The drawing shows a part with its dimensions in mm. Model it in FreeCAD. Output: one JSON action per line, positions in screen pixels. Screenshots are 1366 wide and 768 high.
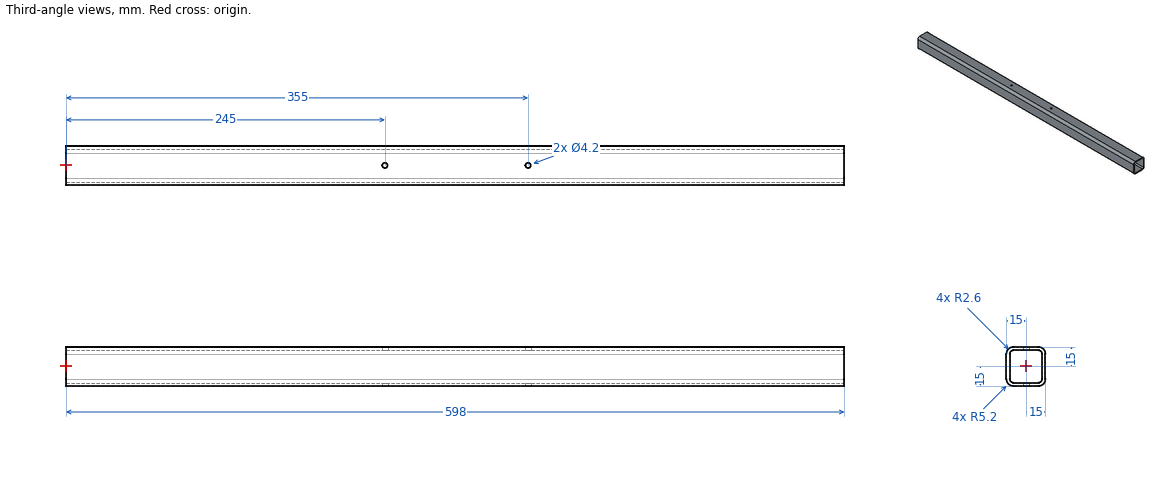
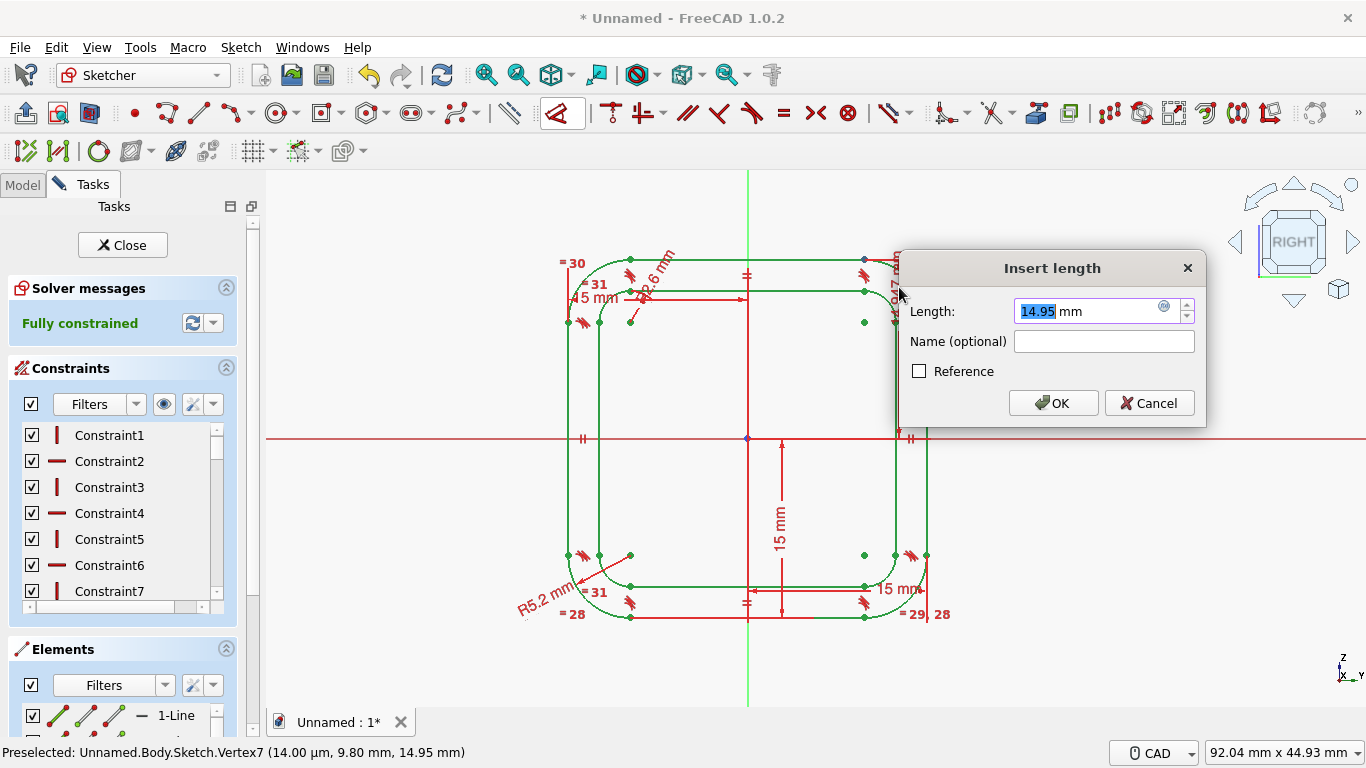
{"action": "type", "text": "15"}
{"action": "key", "text": "Return"}
{"action": "key", "text": "Escape"}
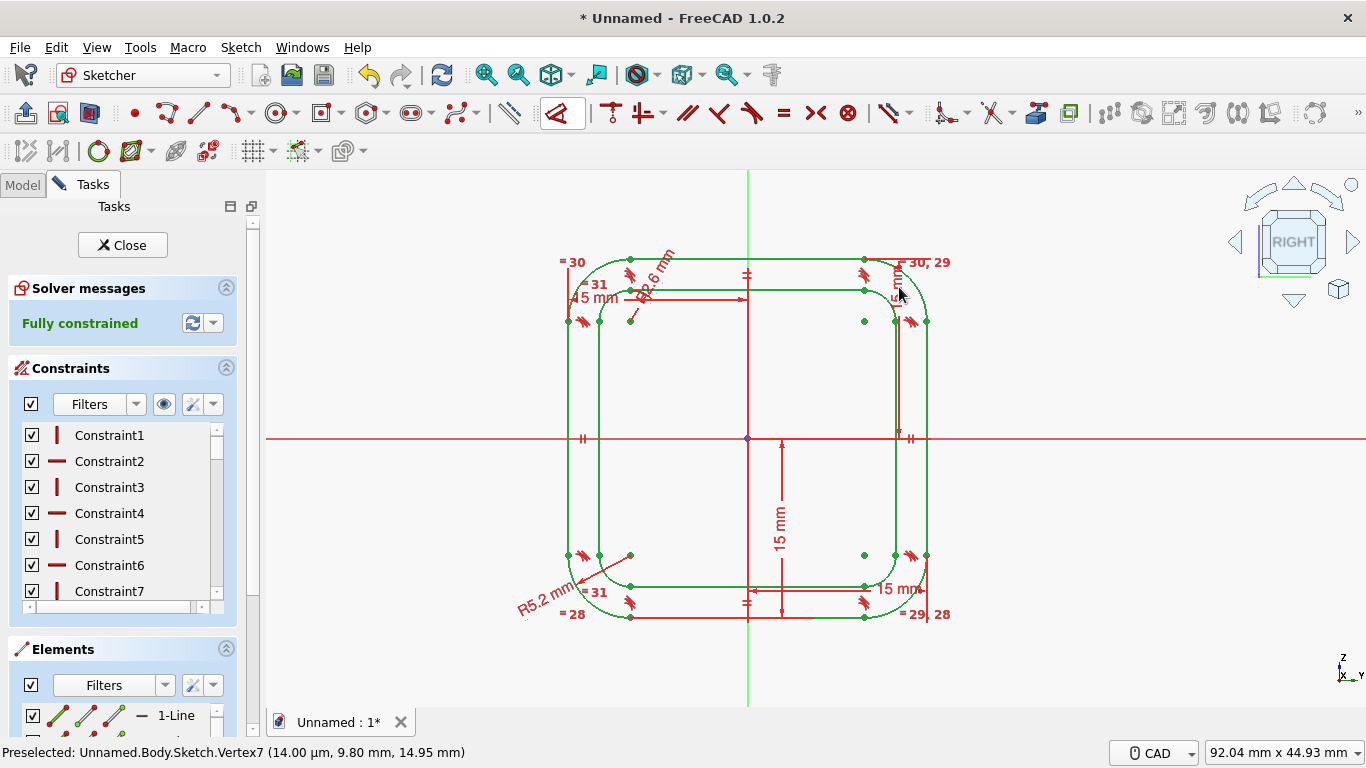
{"action": "left_click", "coordinate": [123, 245]}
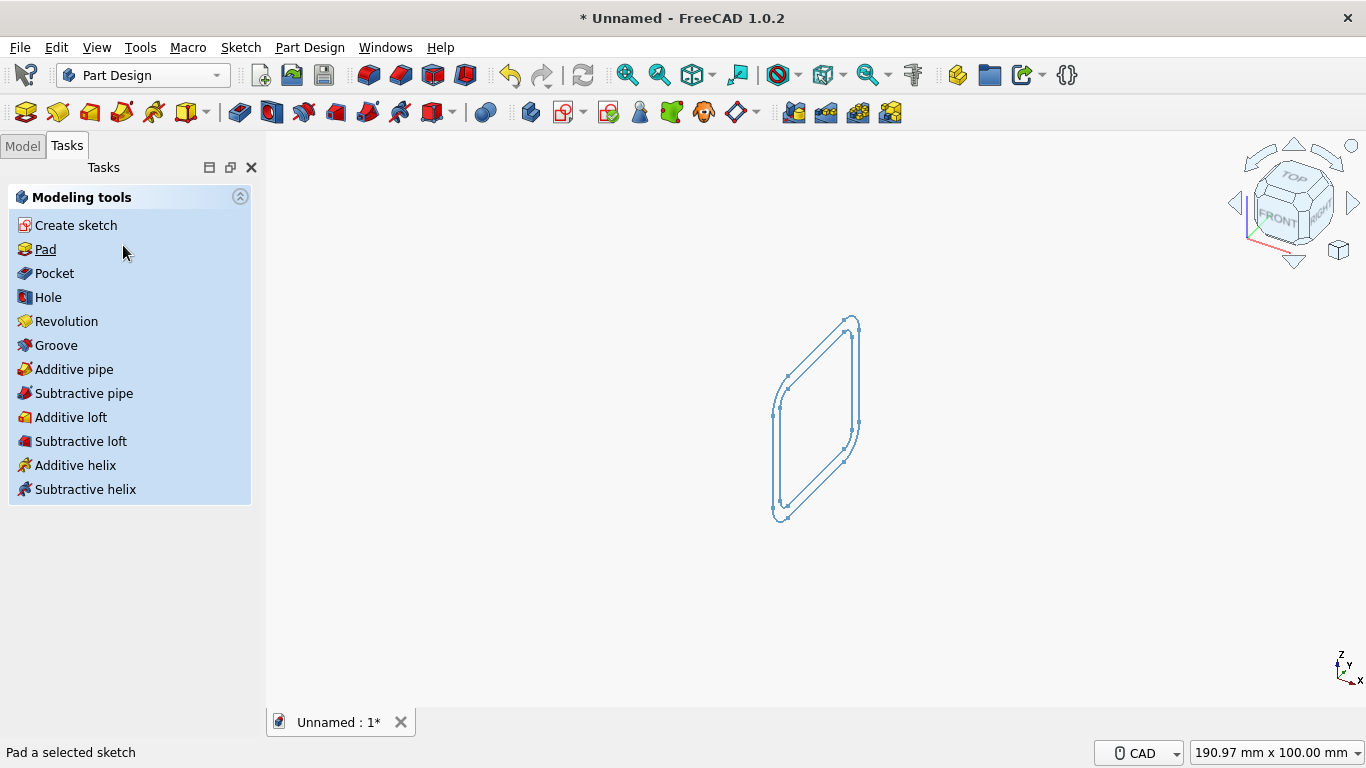
{"action": "left_click", "coordinate": [26, 112]}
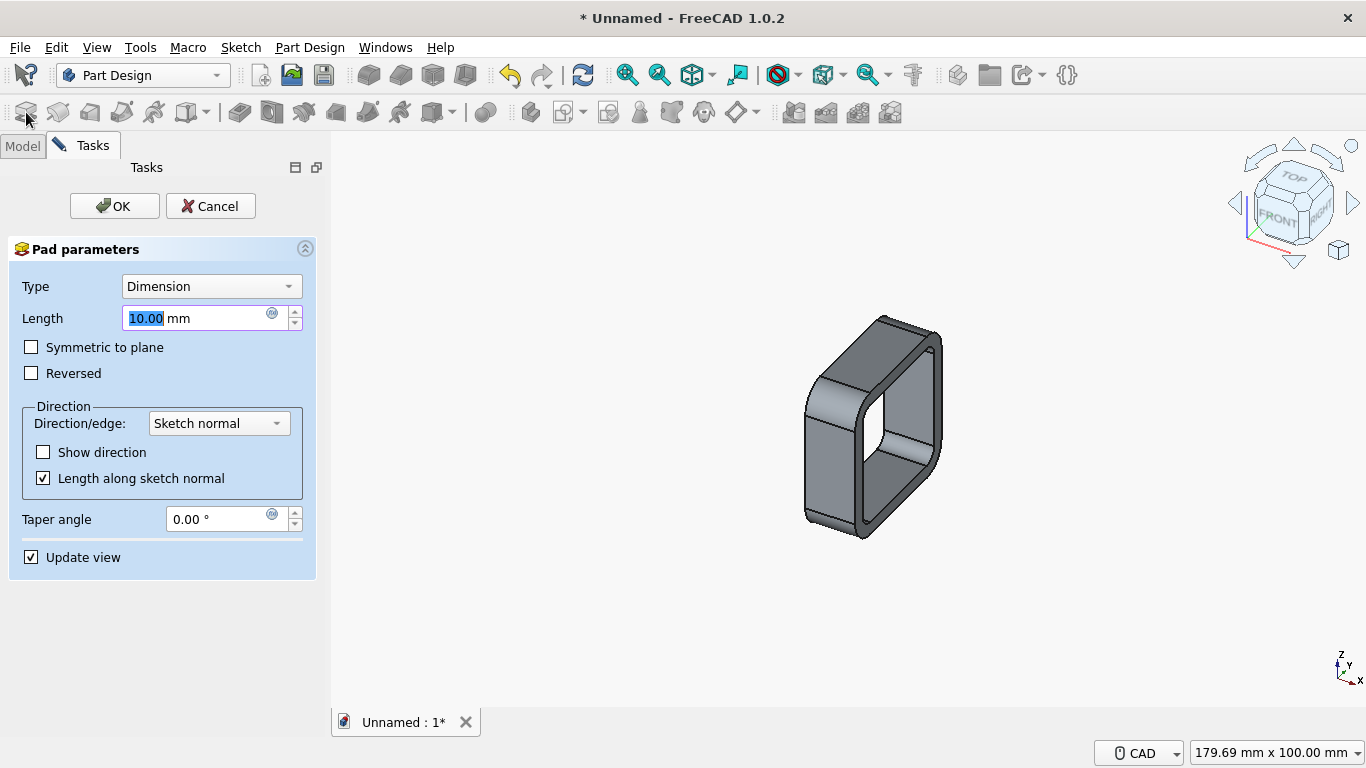
{"action": "type", "text": "598"}
{"action": "key", "text": "Tab"}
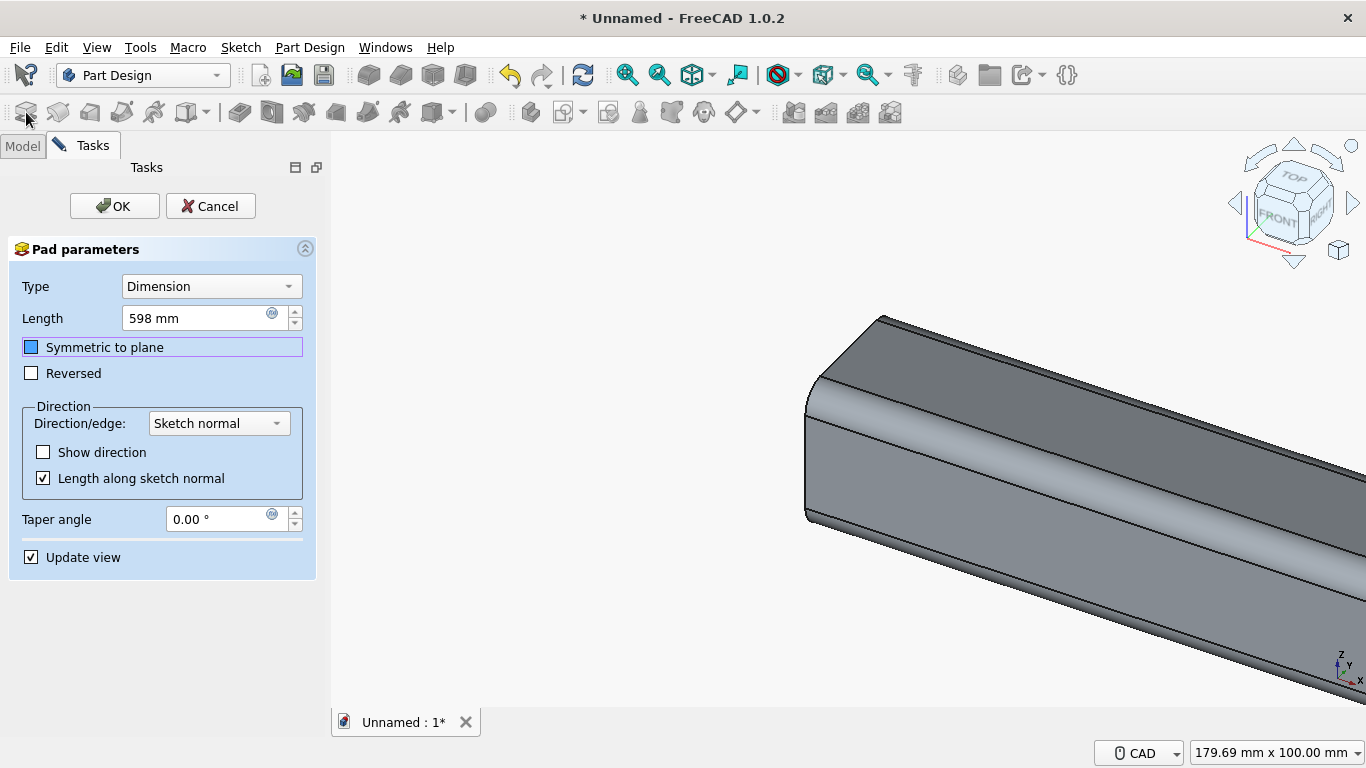
{"action": "left_click", "coordinate": [115, 206]}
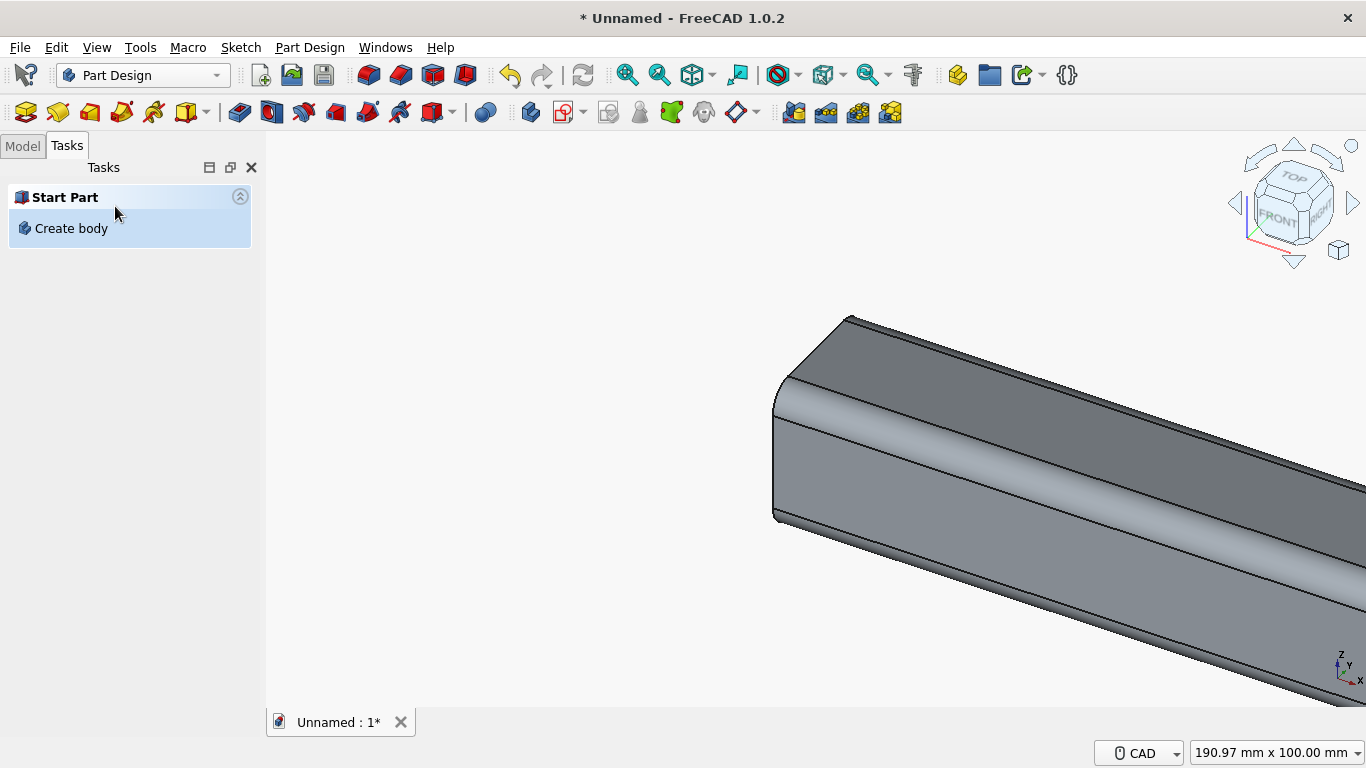
{"action": "left_click", "coordinate": [628, 76]}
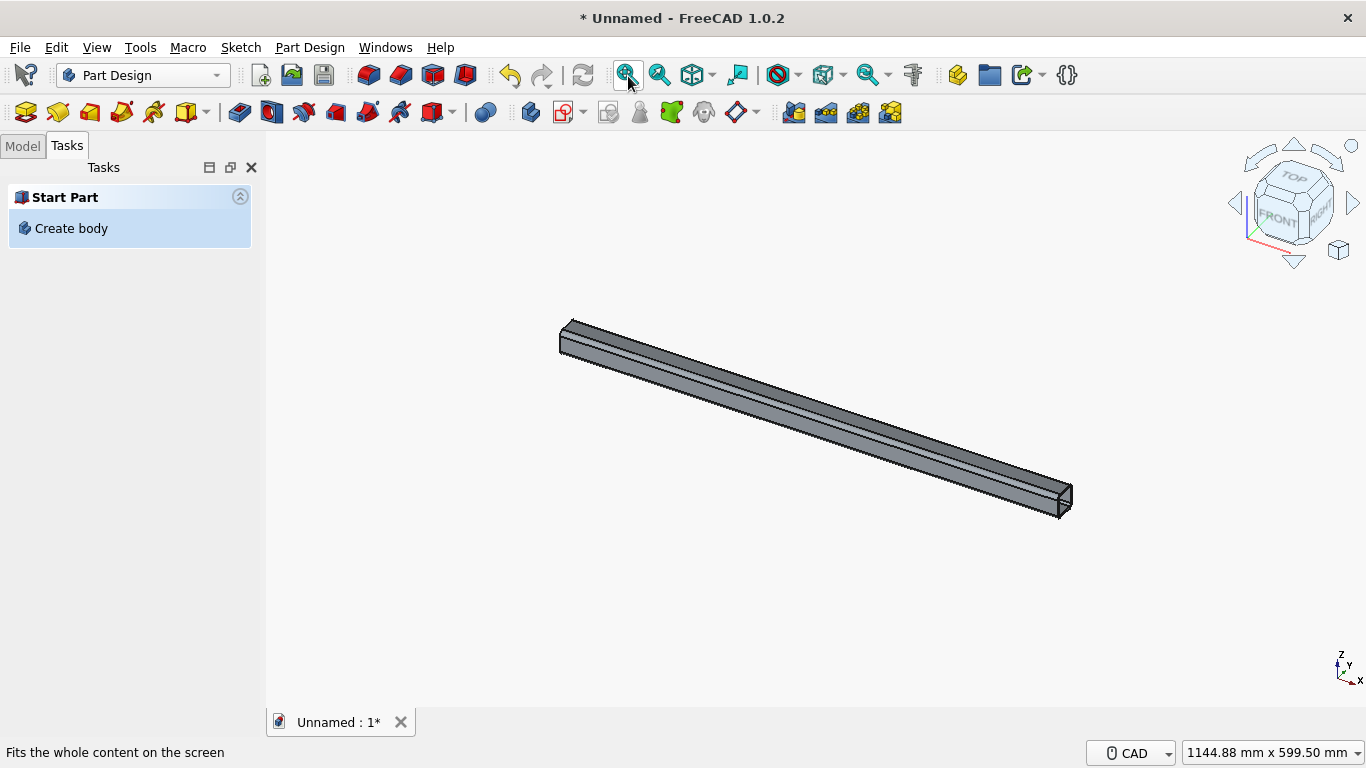
{"action": "key", "text": "0"}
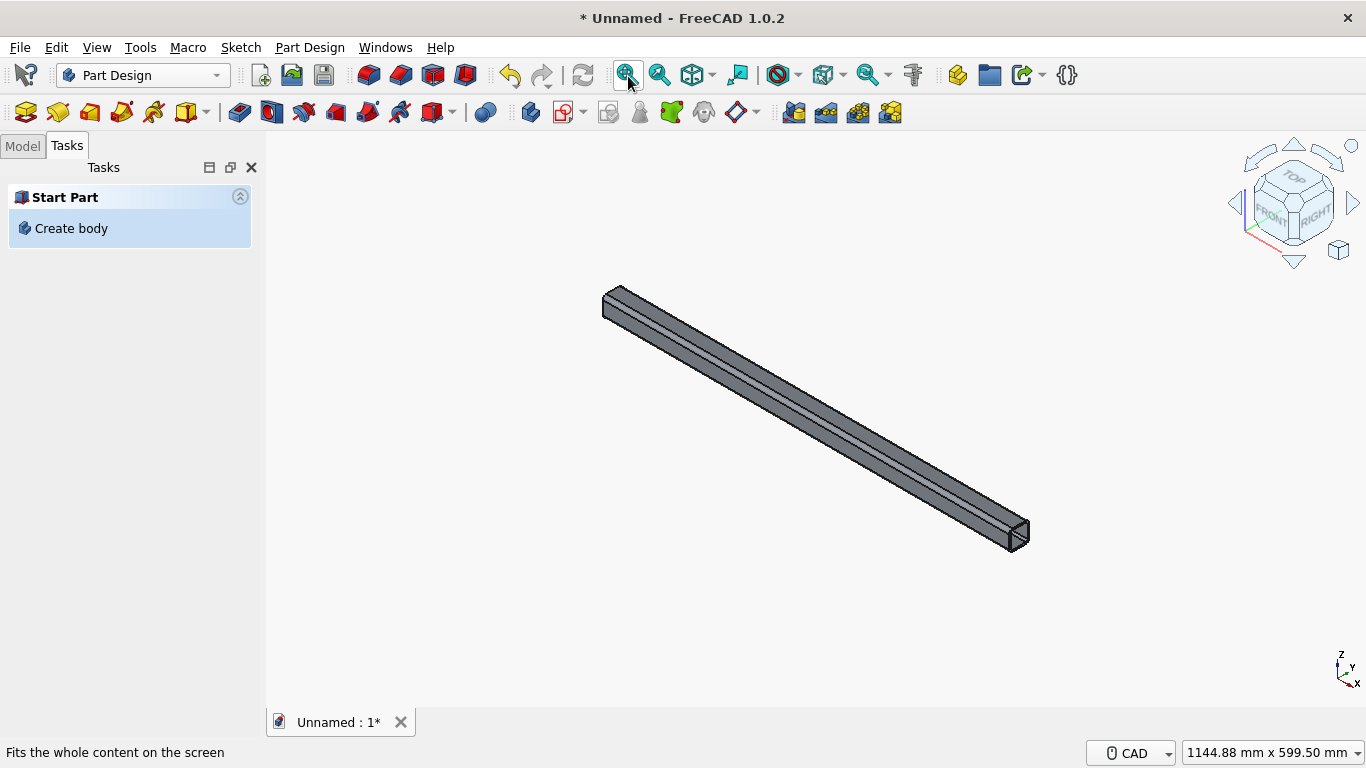
{"action": "key", "text": "2"}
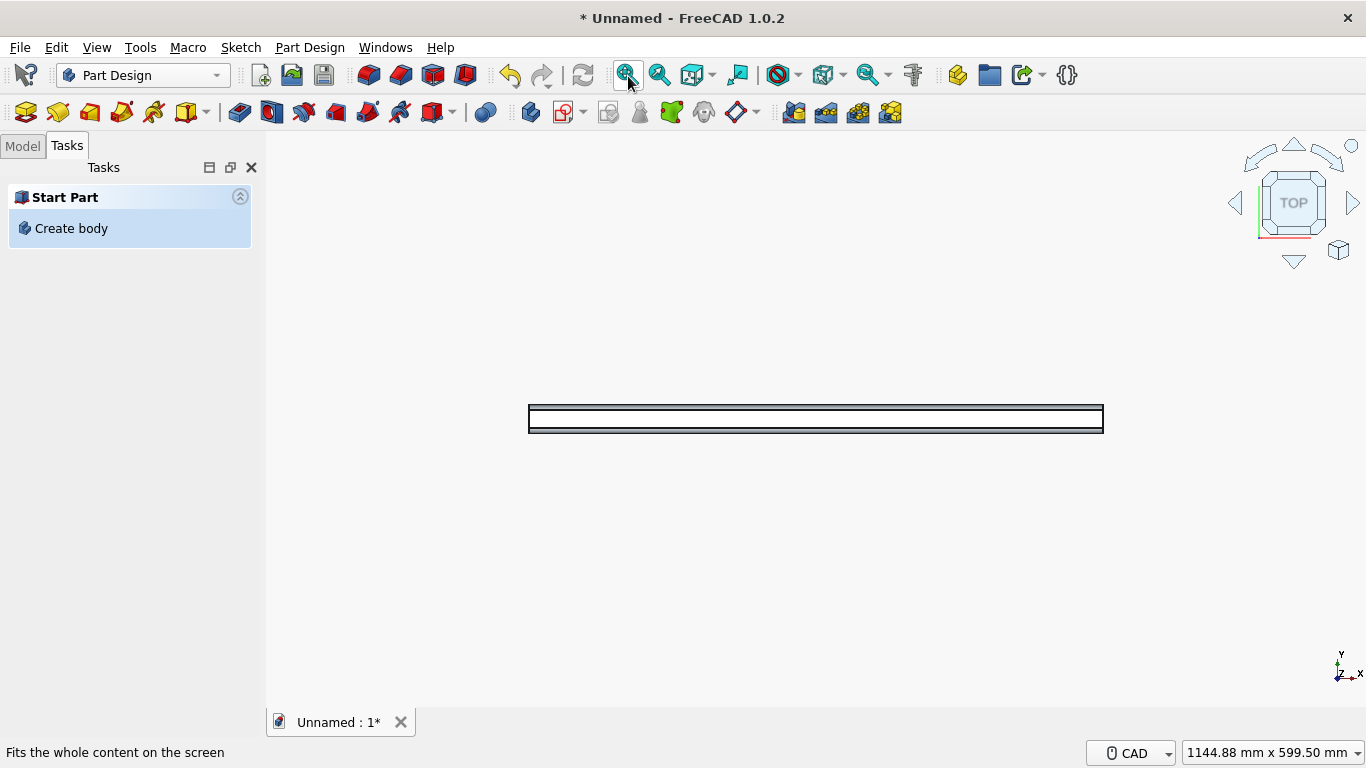
{"action": "left_click", "coordinate": [816, 418]}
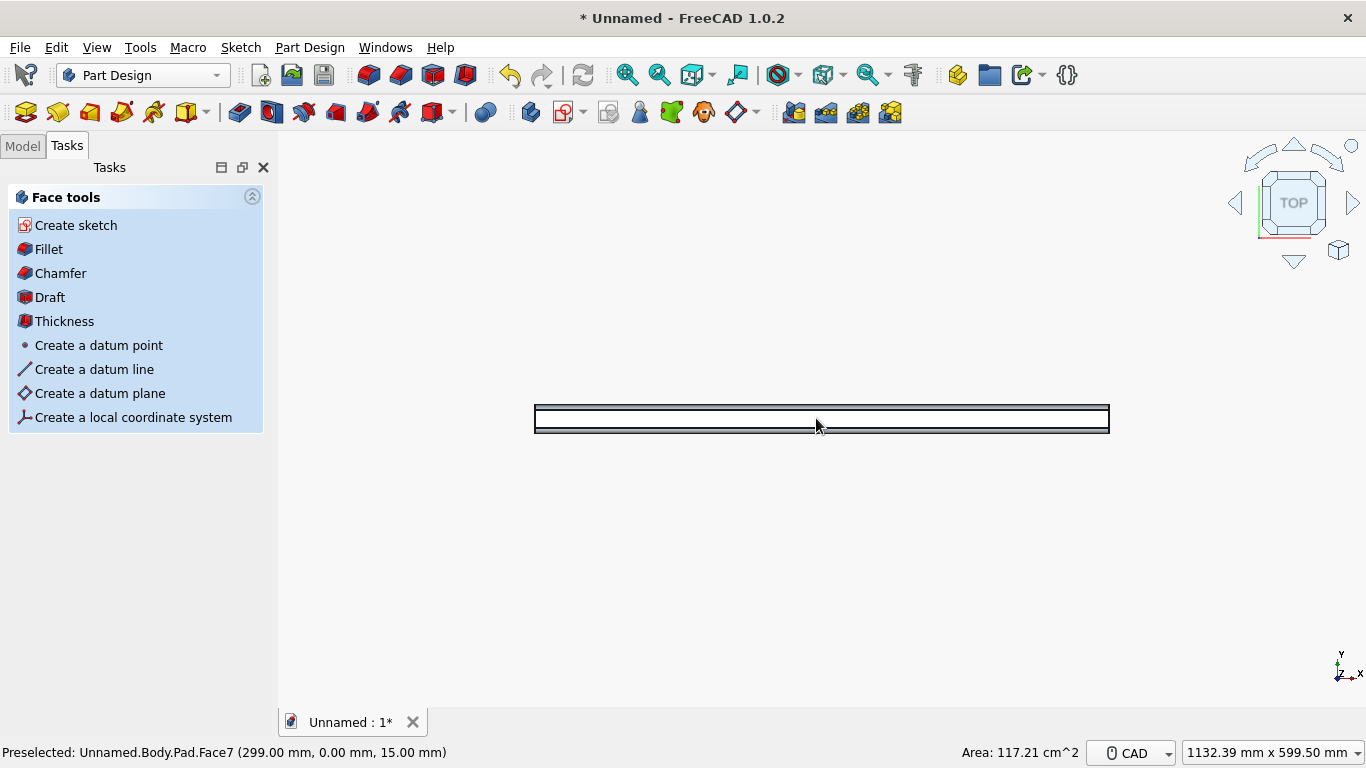
{"action": "left_click", "coordinate": [564, 112]}